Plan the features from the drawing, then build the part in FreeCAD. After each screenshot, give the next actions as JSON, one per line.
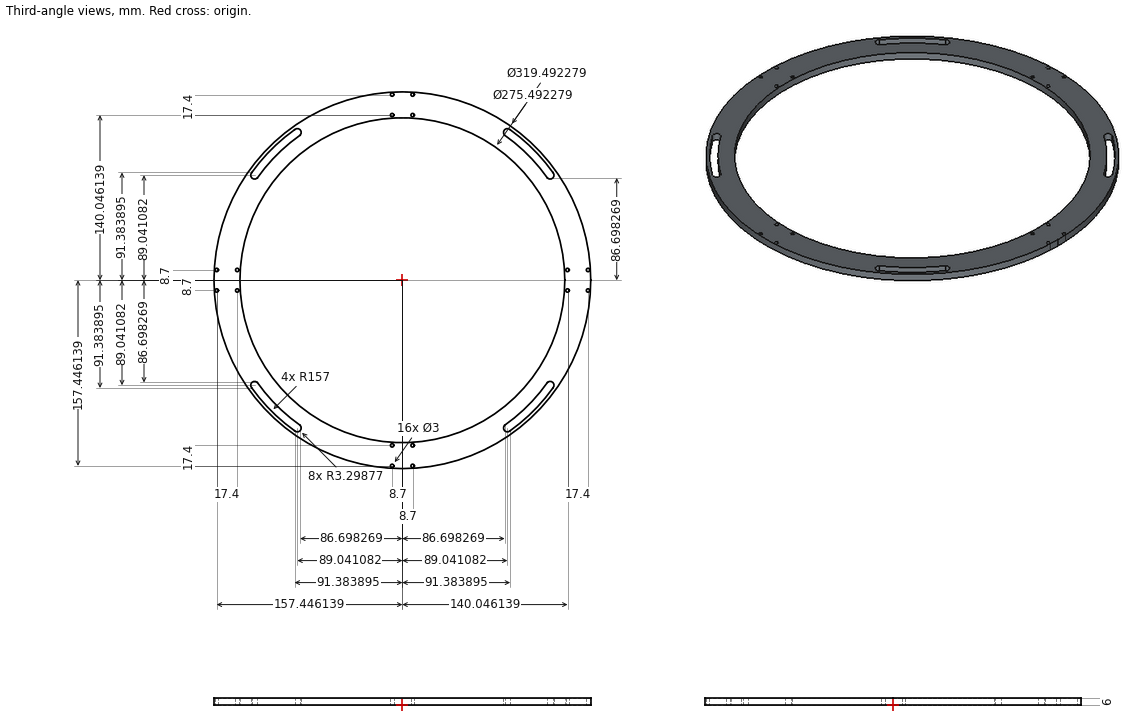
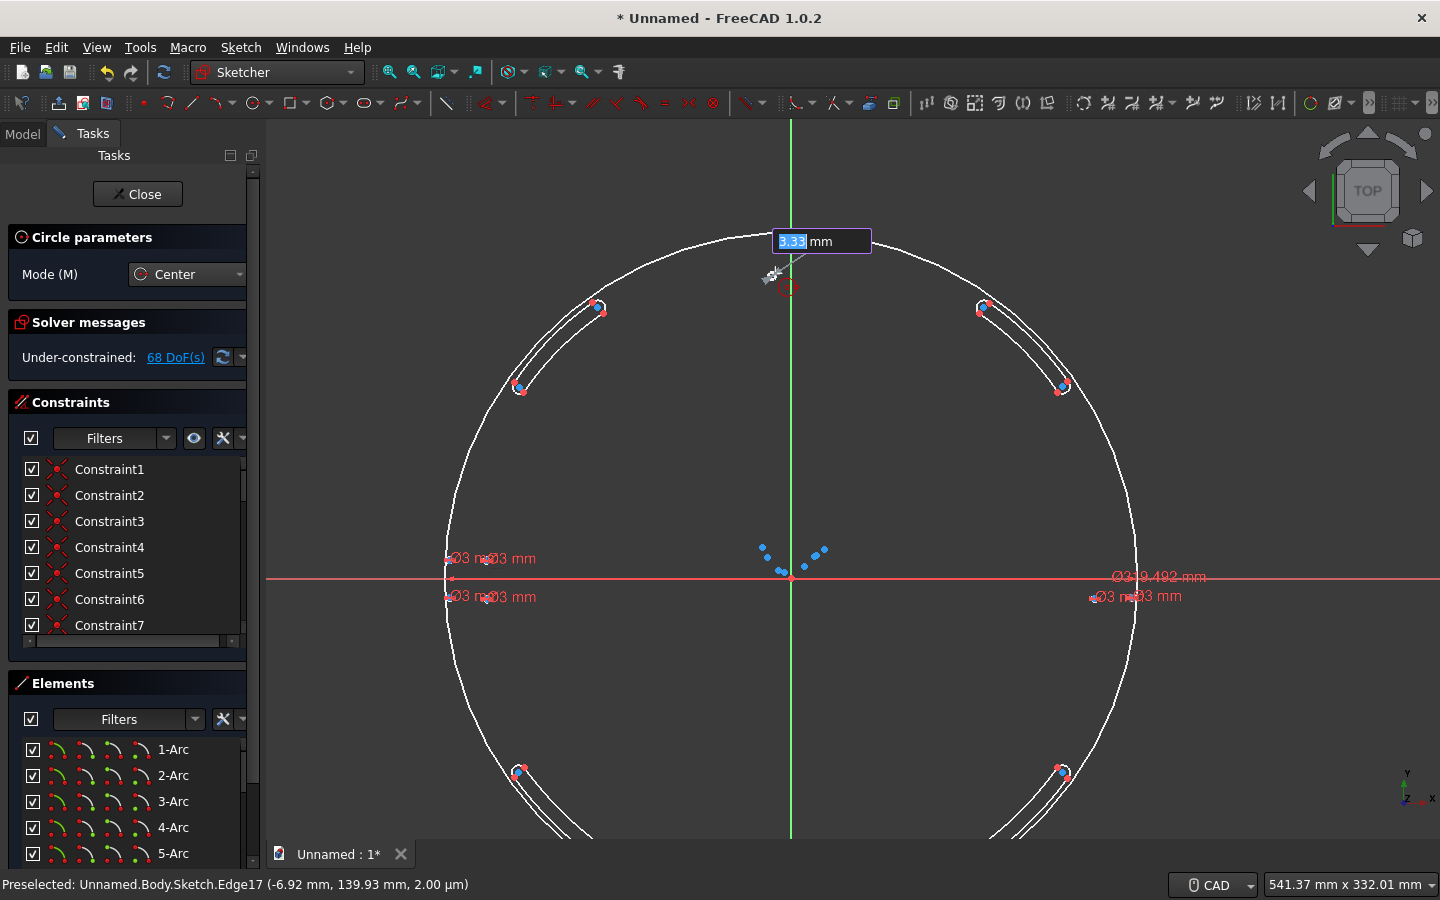
{"action": "type", "text": "3"}
{"action": "key", "text": "Return"}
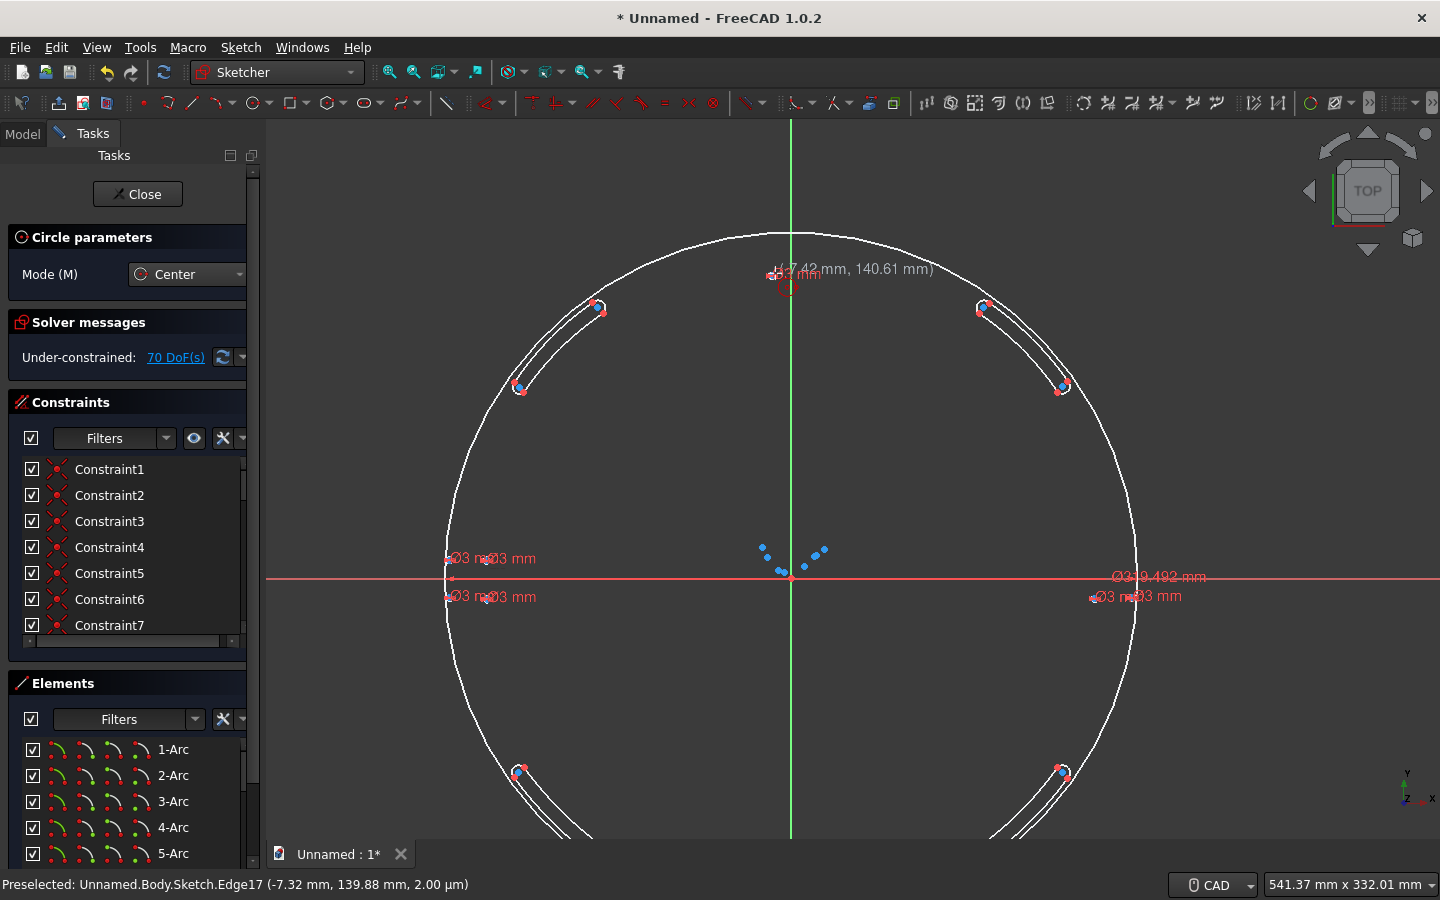
{"action": "scroll", "coordinate": [772, 237], "scroll_direction": "up", "scroll_amount": 10}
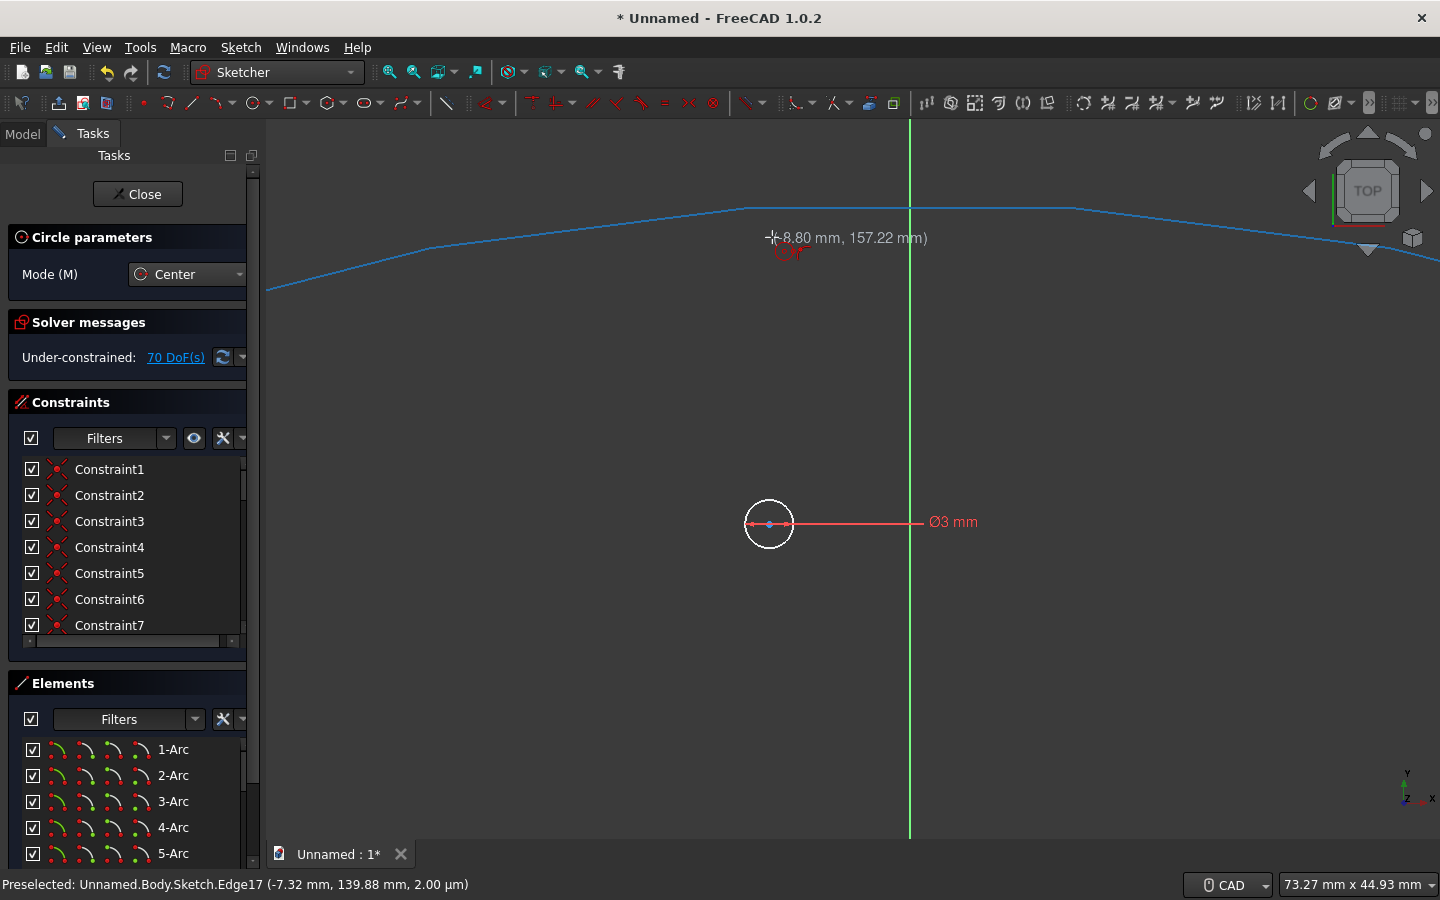
{"action": "left_click", "coordinate": [771, 240]}
{"action": "mouse_move", "coordinate": [788, 223]}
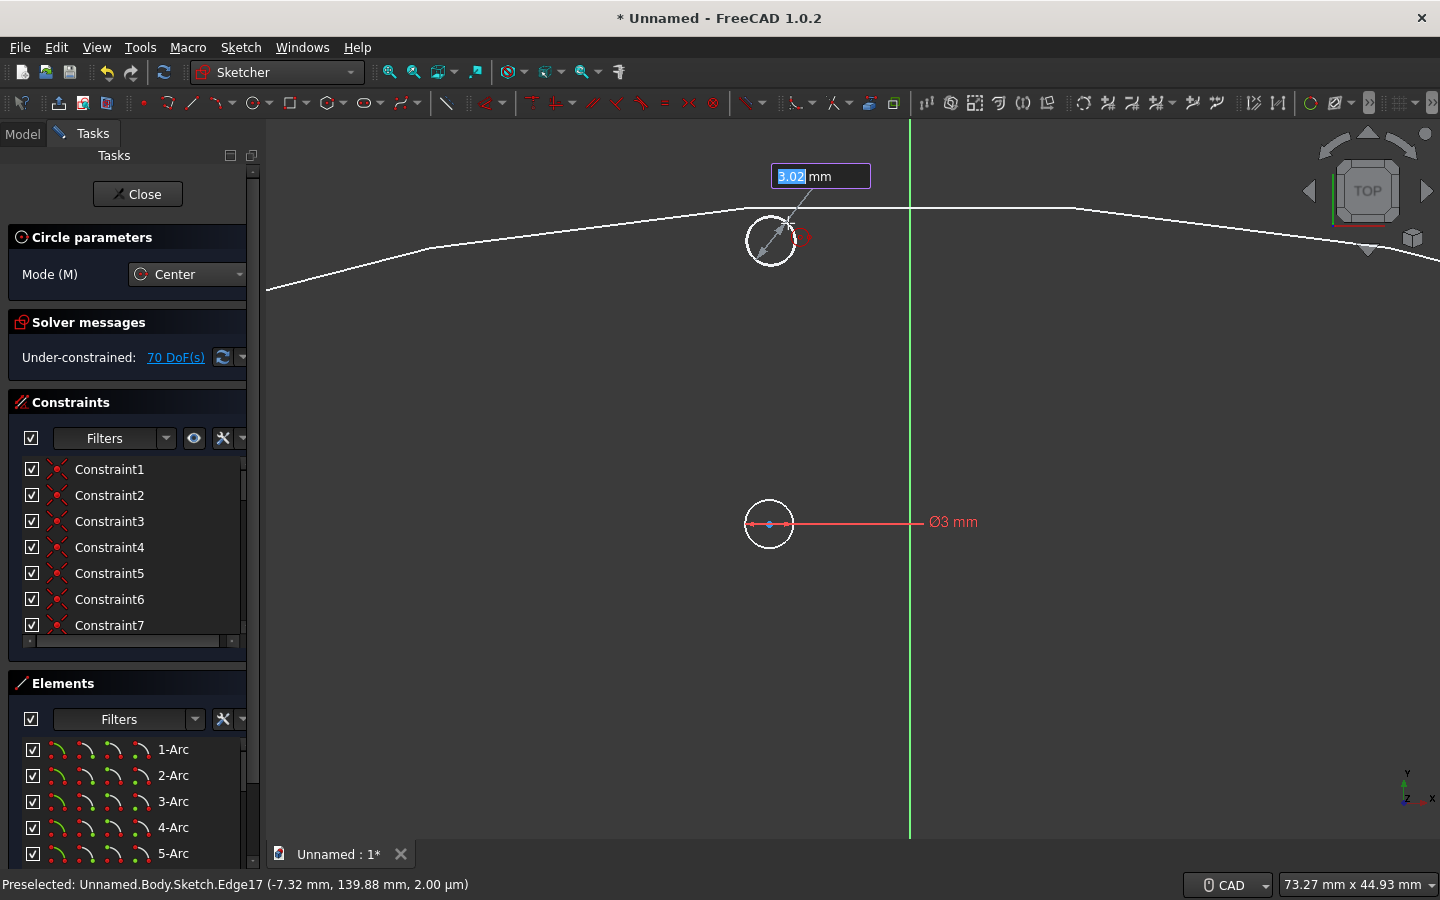
{"action": "type", "text": "3"}
{"action": "key", "text": "Return"}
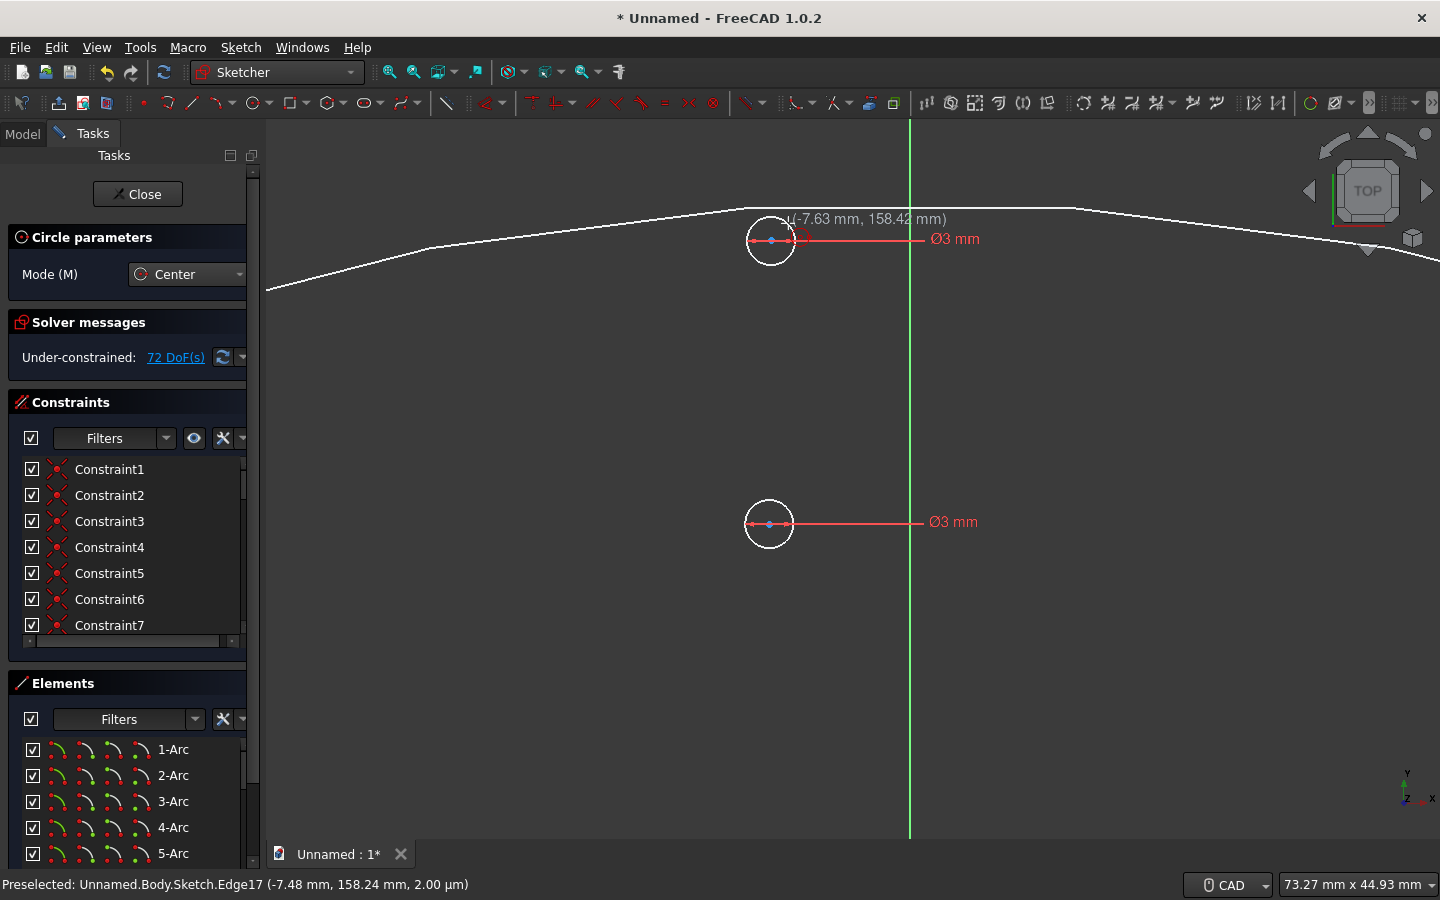
{"action": "scroll", "coordinate": [772, 251], "scroll_direction": "down", "scroll_amount": 12}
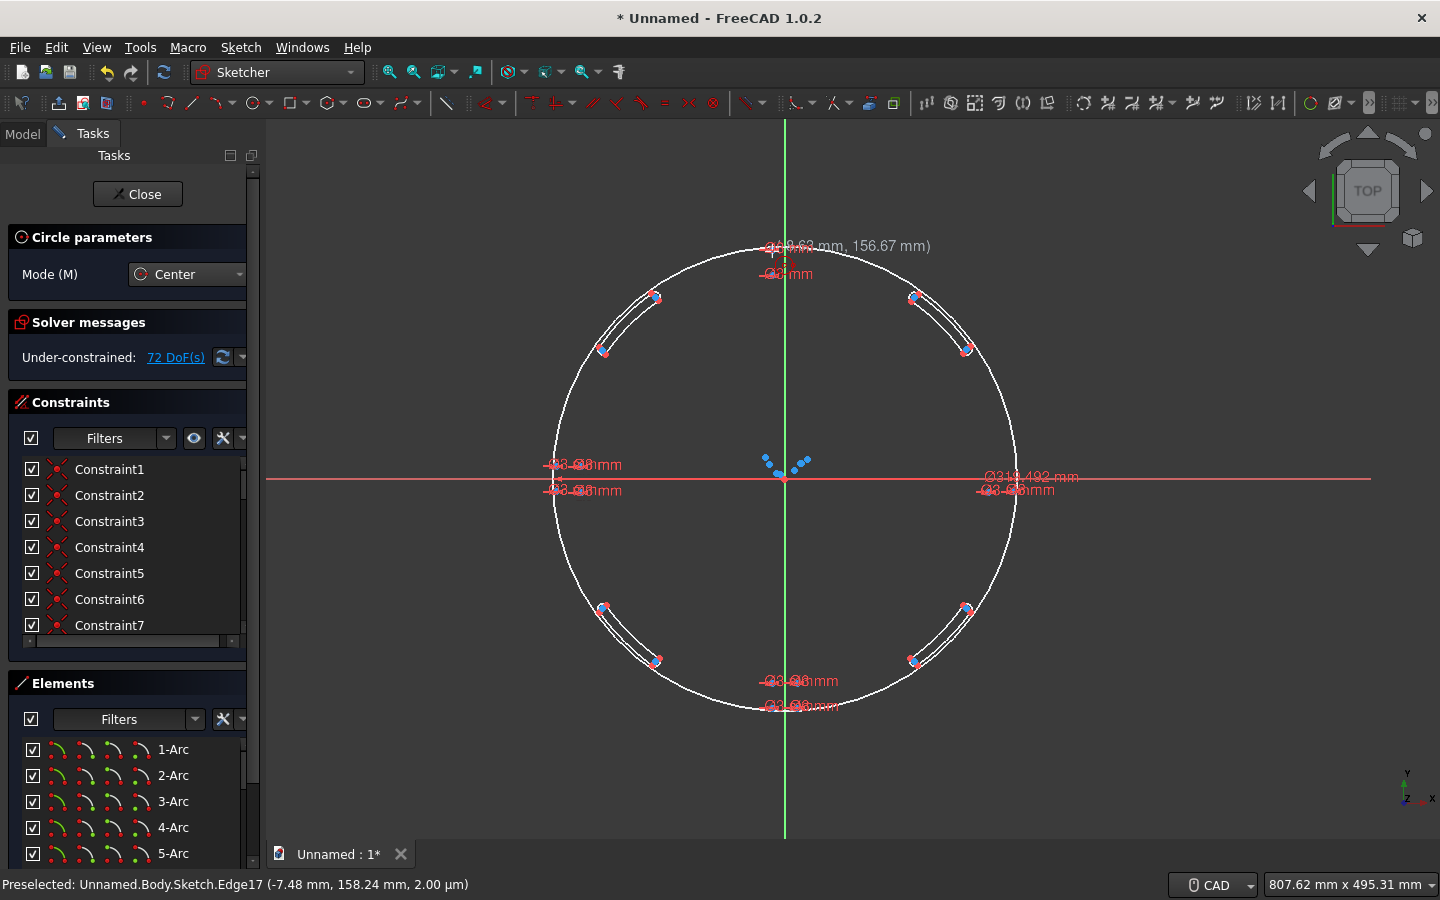
{"action": "left_click", "coordinate": [785, 479]}
{"action": "mouse_move", "coordinate": [927, 337]}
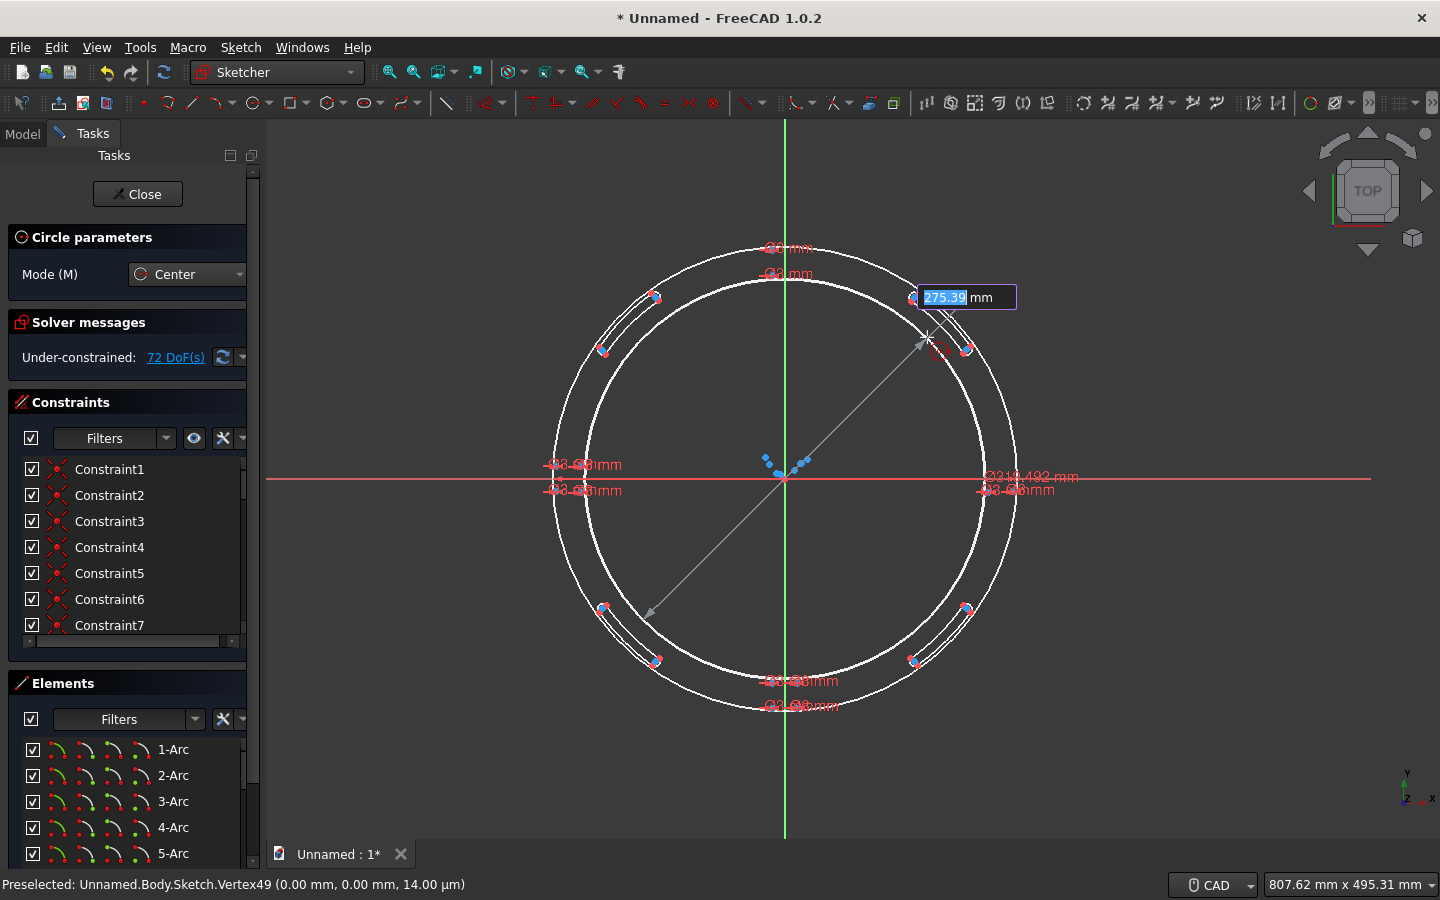
{"action": "type", "text": "275.492279"}
{"action": "key", "text": "Return"}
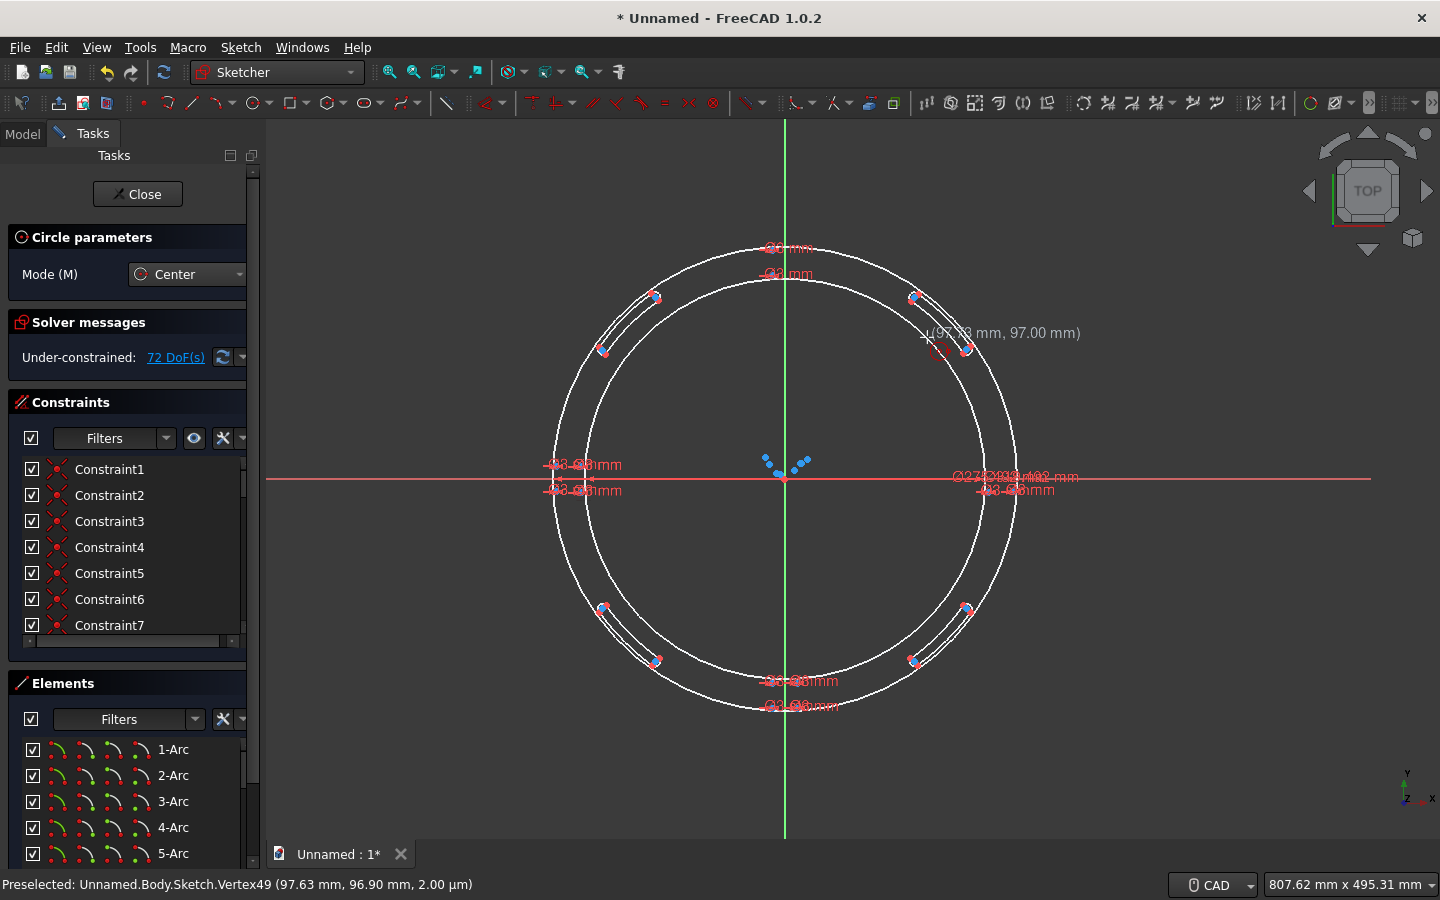
{"action": "scroll", "coordinate": [989, 466], "scroll_direction": "up", "scroll_amount": 12}